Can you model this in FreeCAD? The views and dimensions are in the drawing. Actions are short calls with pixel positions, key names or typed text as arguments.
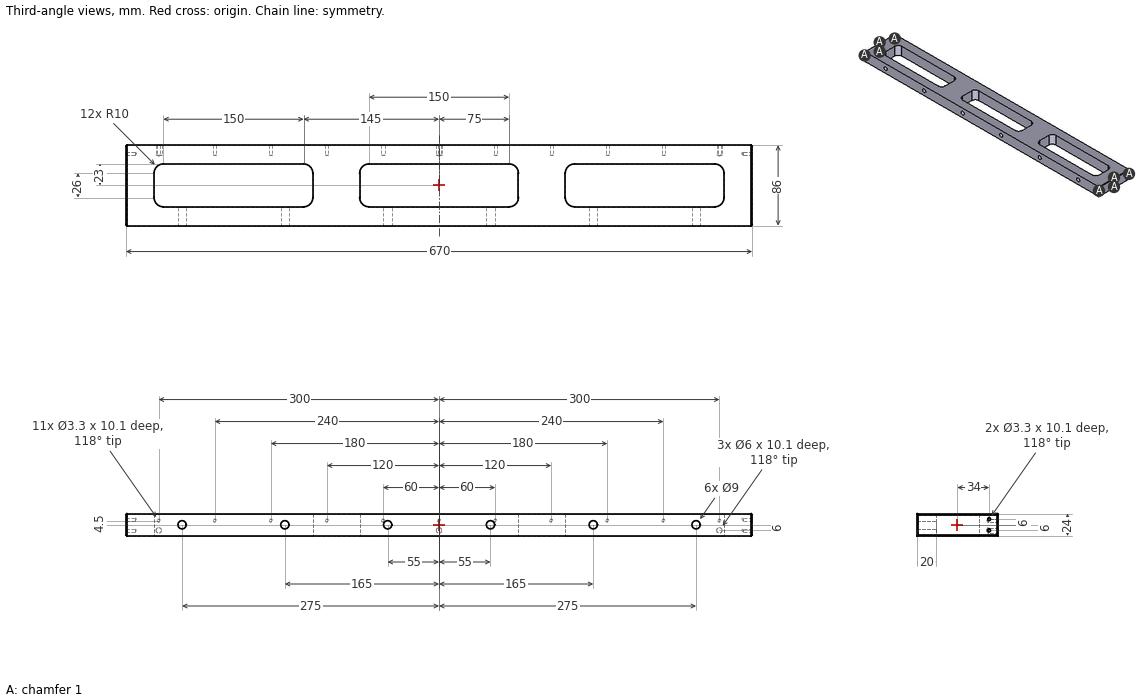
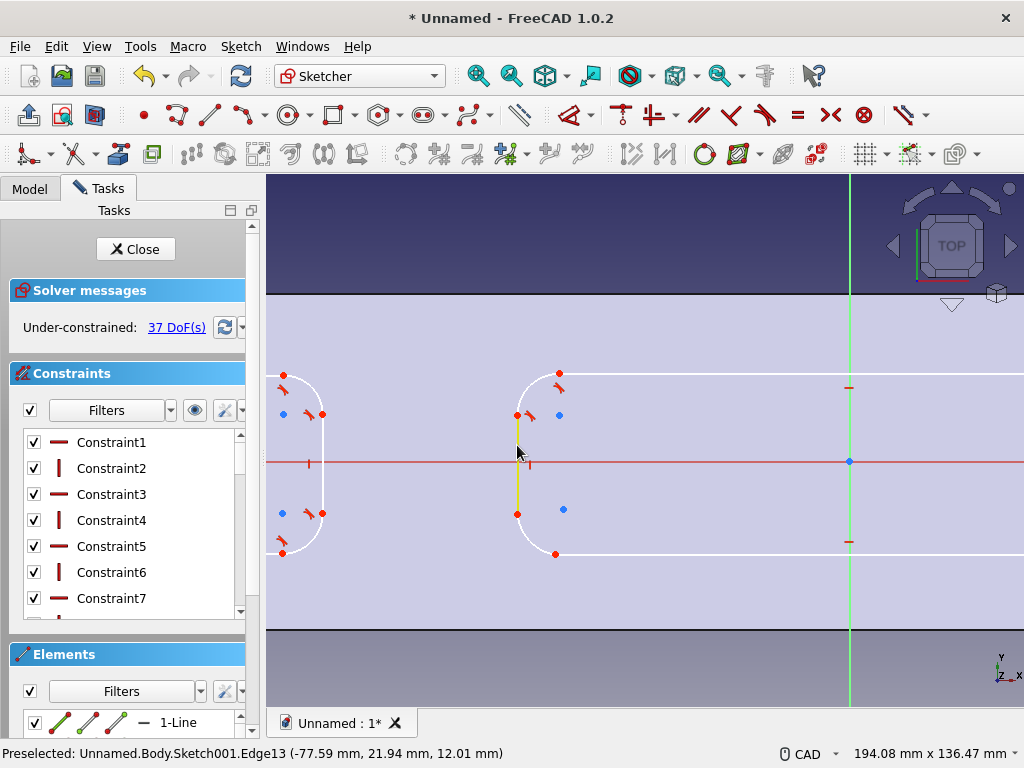
click(518, 445)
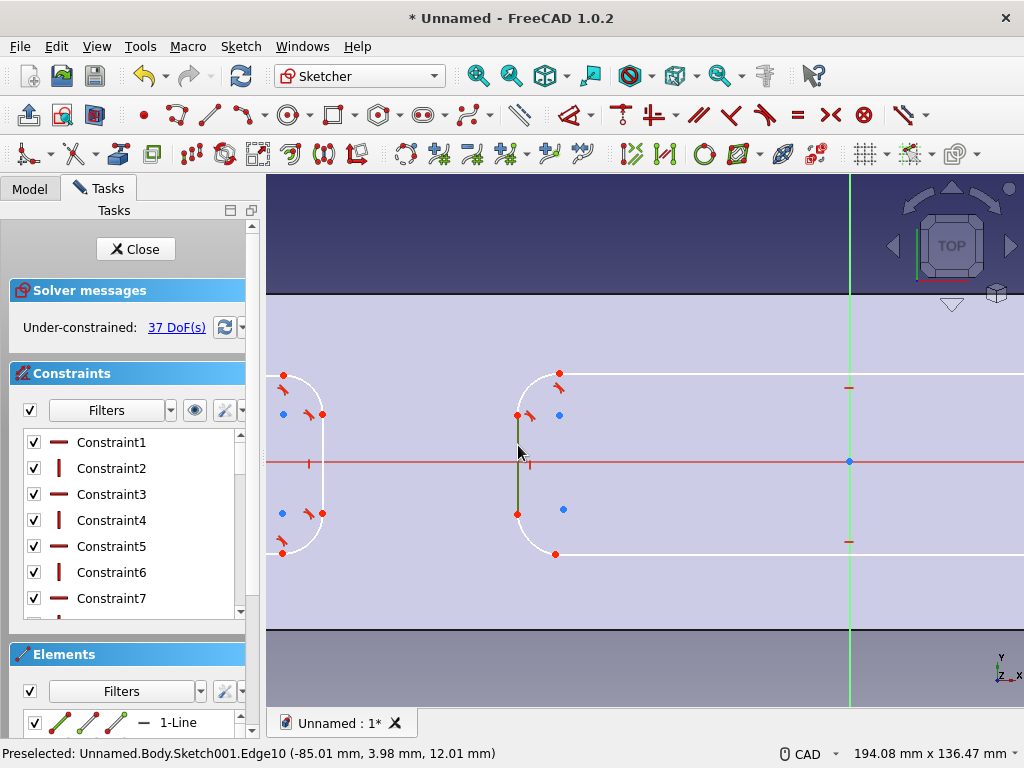
click(523, 531)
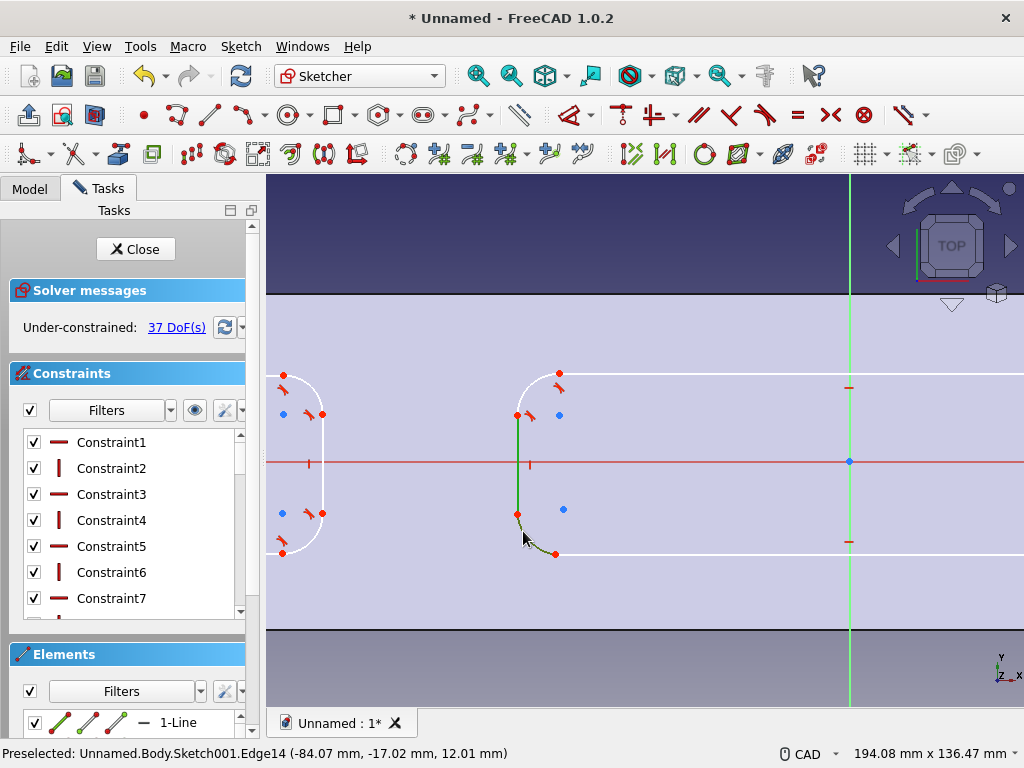
key(t)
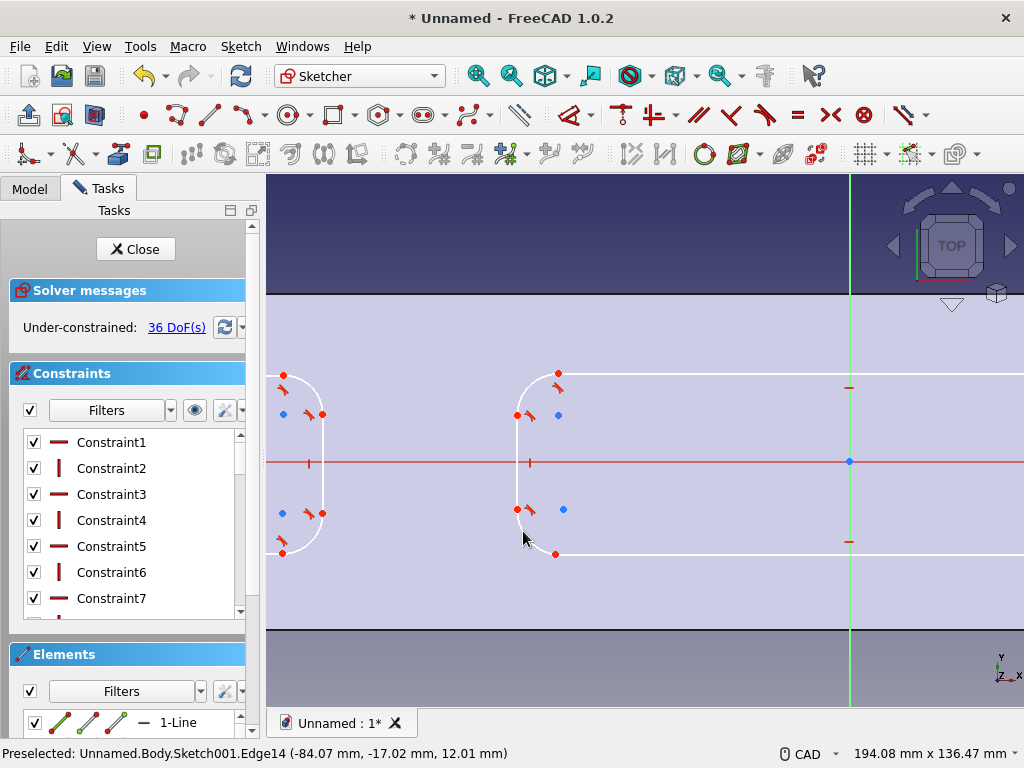
scroll(522, 436, down, 9)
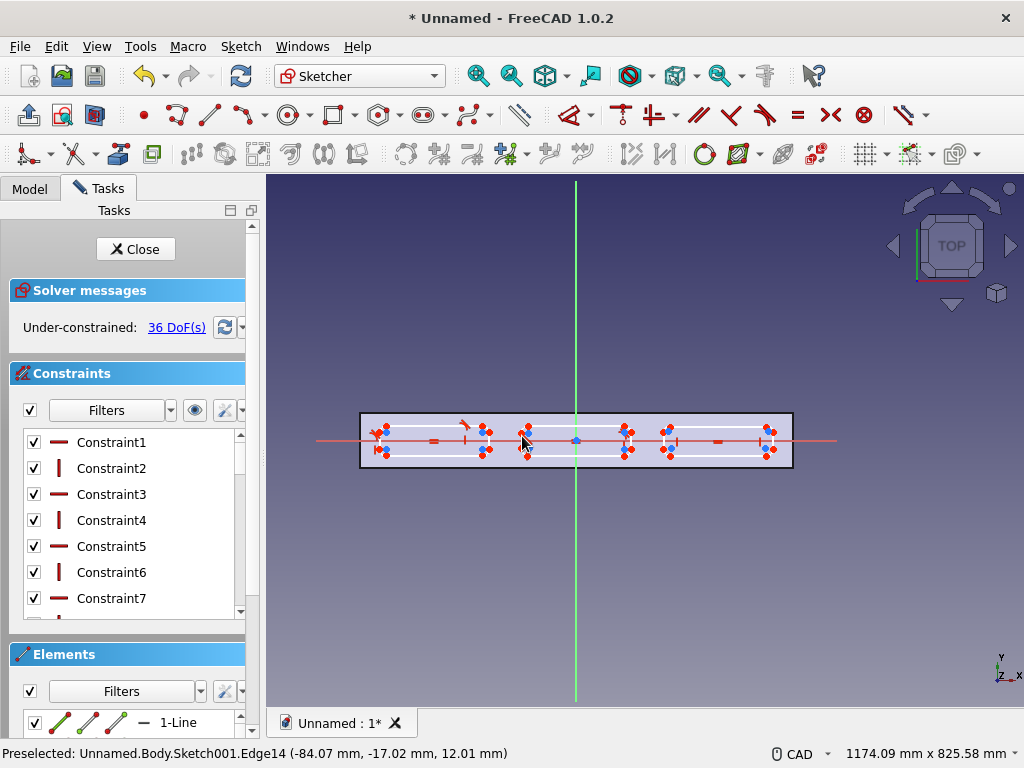
click(557, 456)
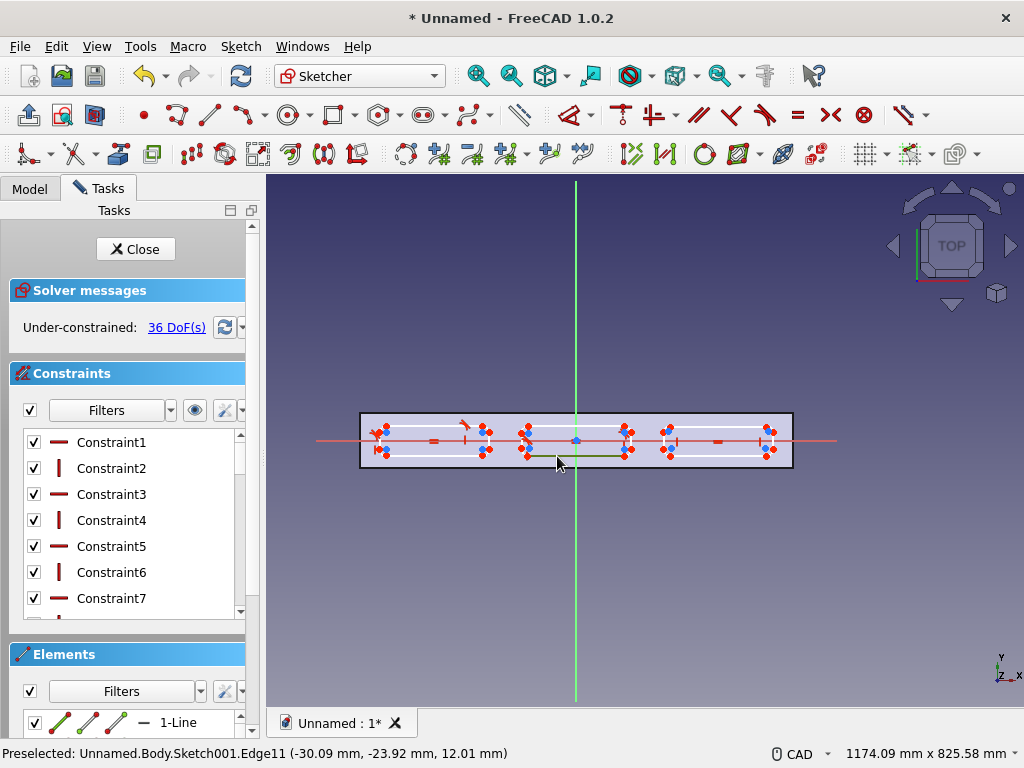
scroll(523, 453, up, 5)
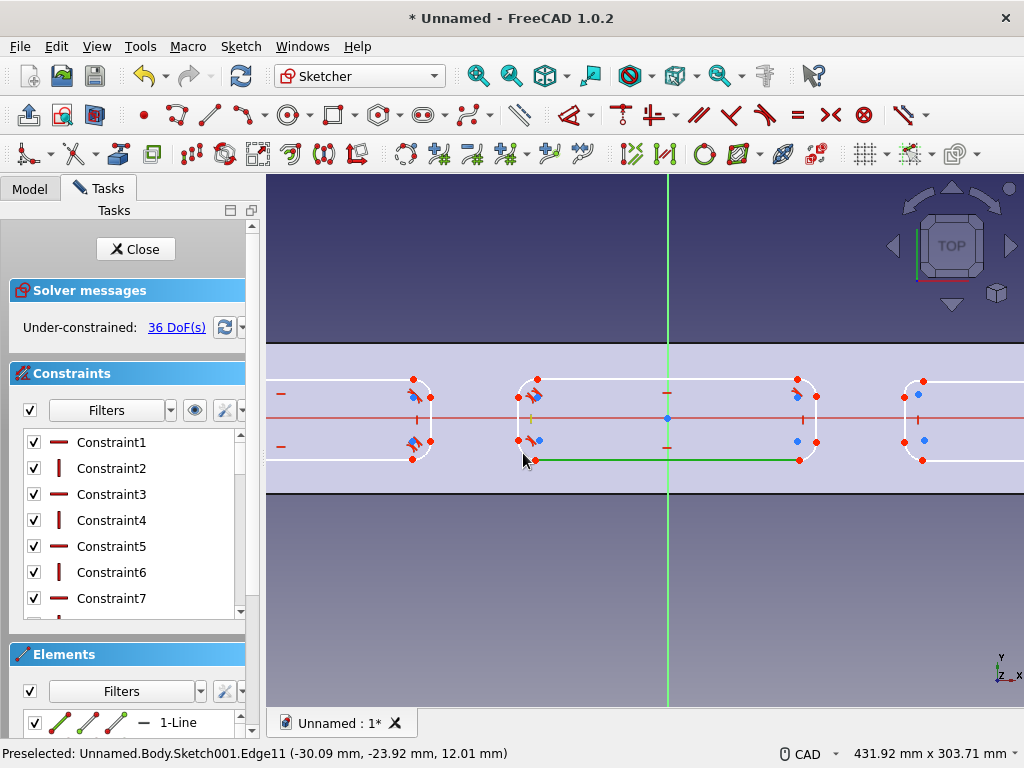
click(523, 453)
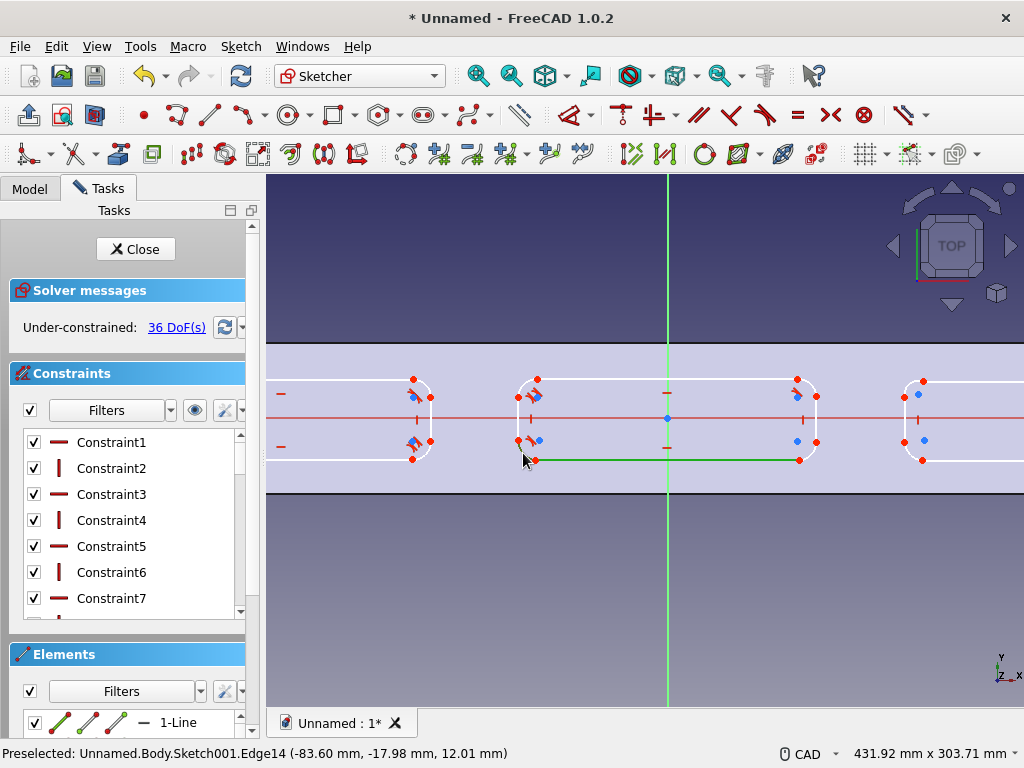
key(t)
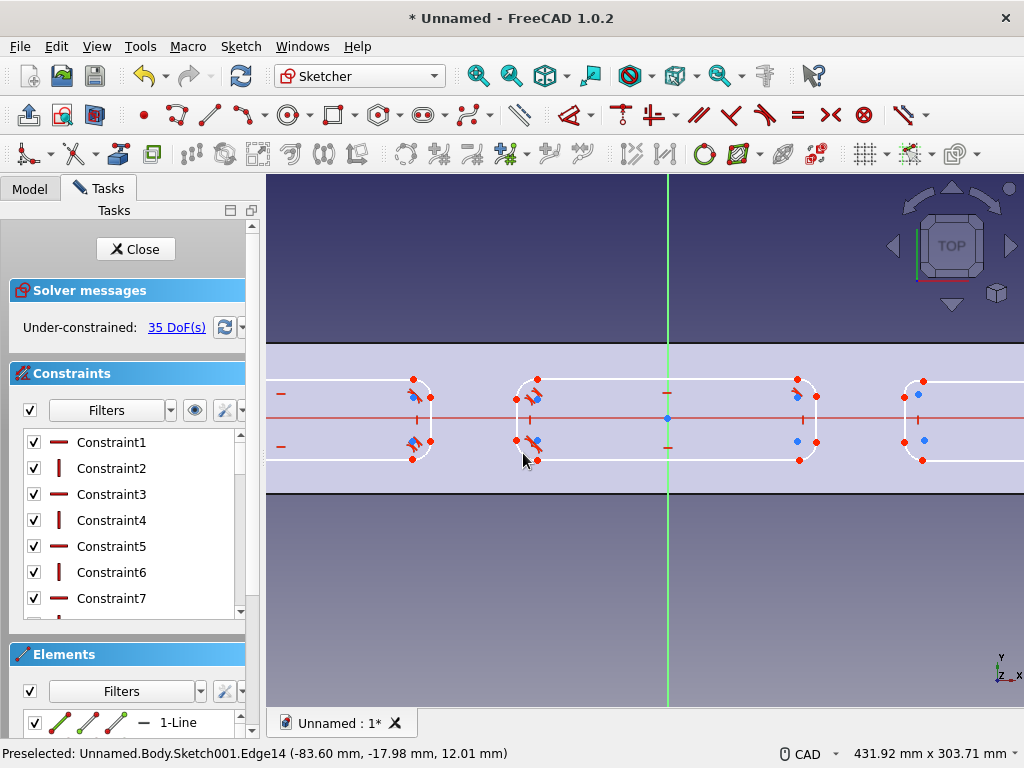
click(616, 460)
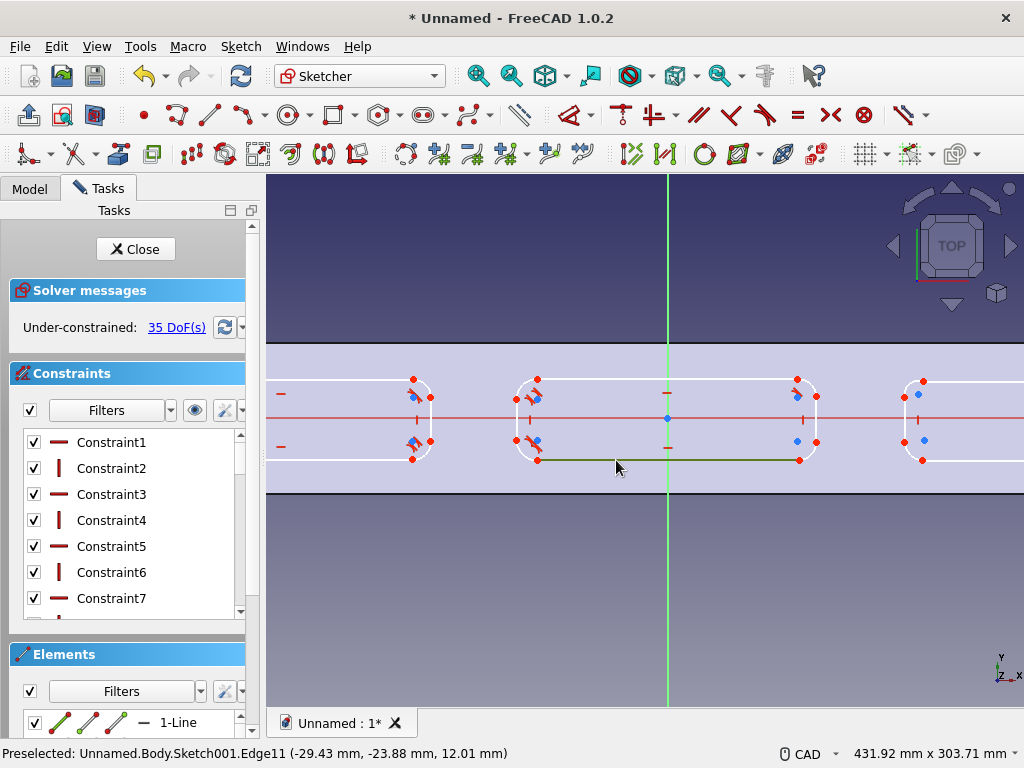
click(811, 454)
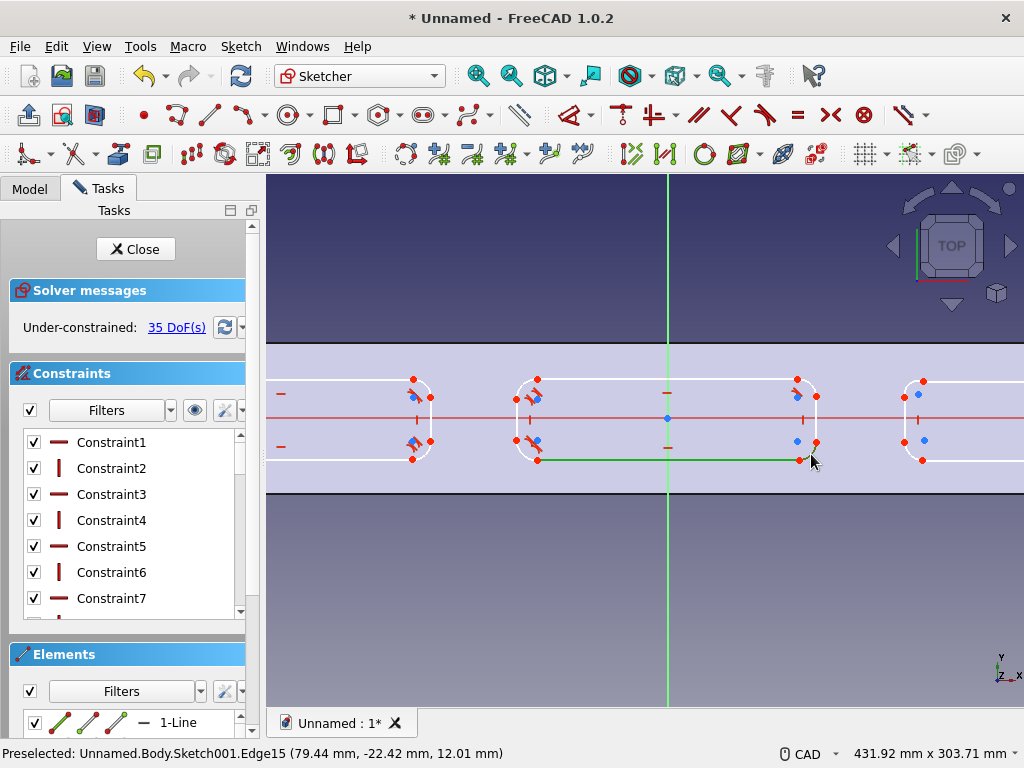
key(t)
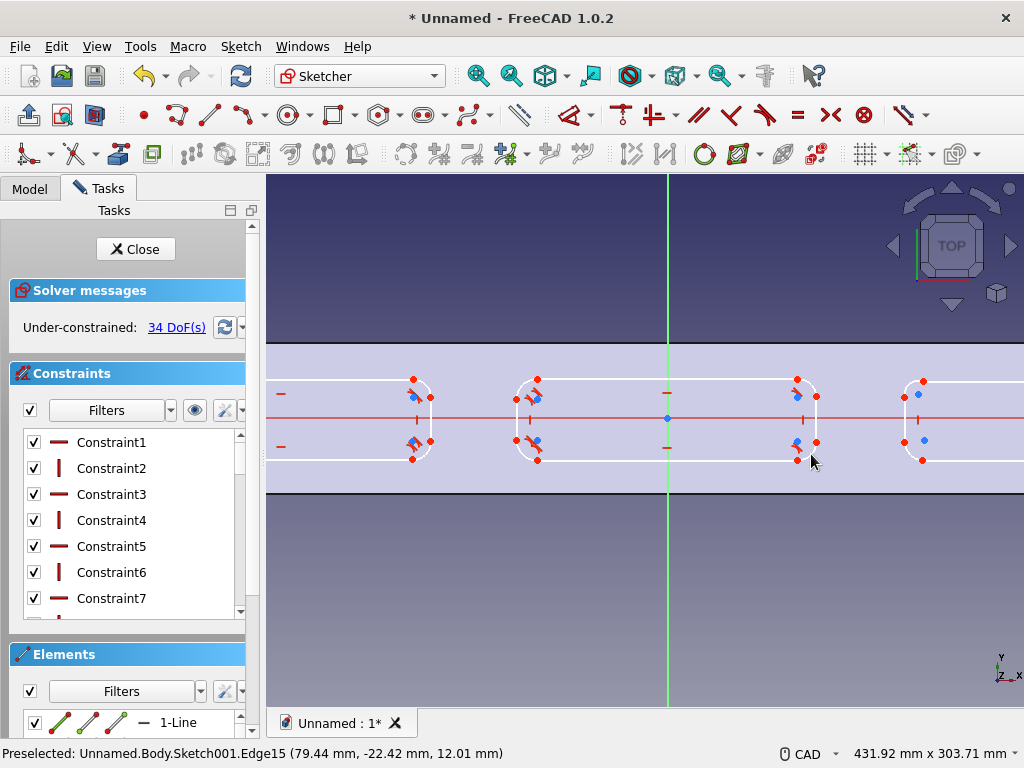
scroll(816, 429, up, 2)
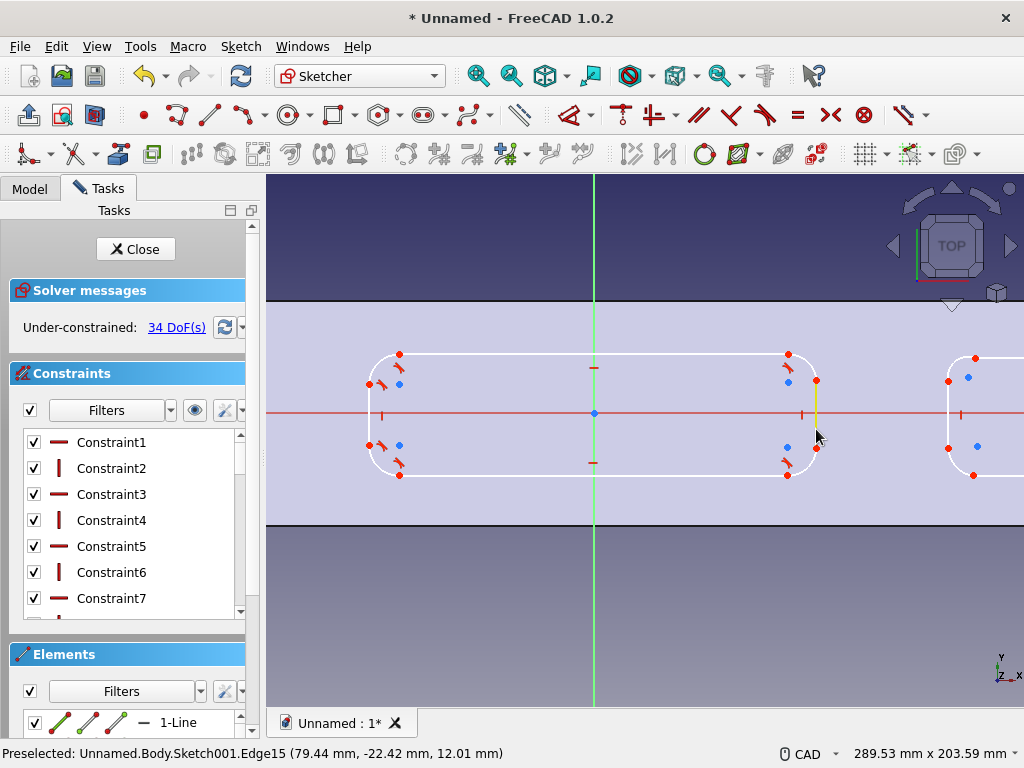
click(816, 428)